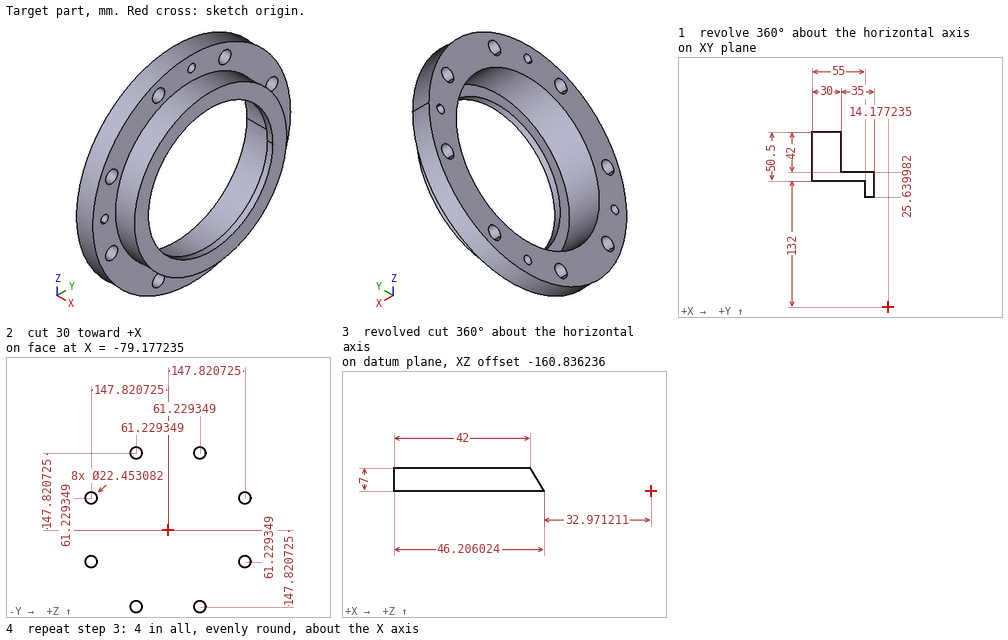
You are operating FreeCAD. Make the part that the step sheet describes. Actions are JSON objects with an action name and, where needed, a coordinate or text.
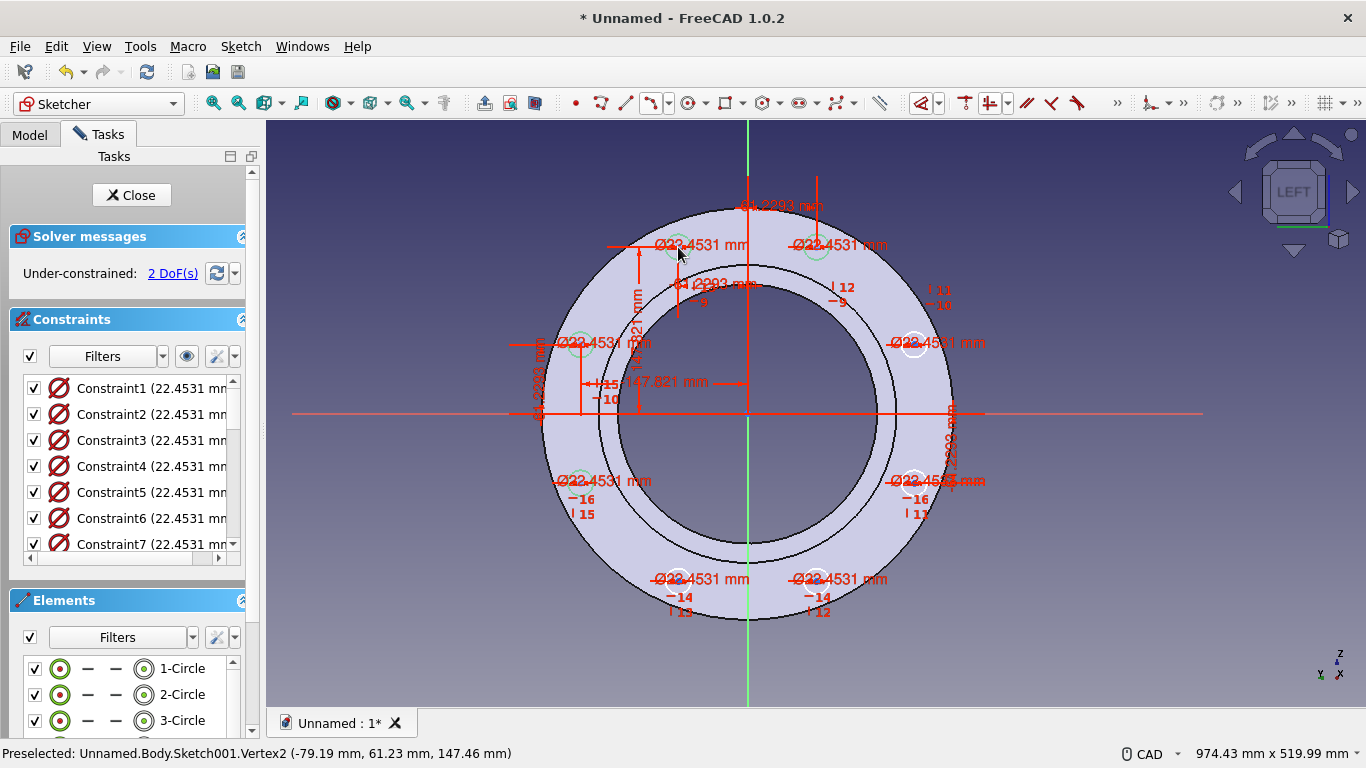
{"action": "left_click", "coordinate": [914, 345]}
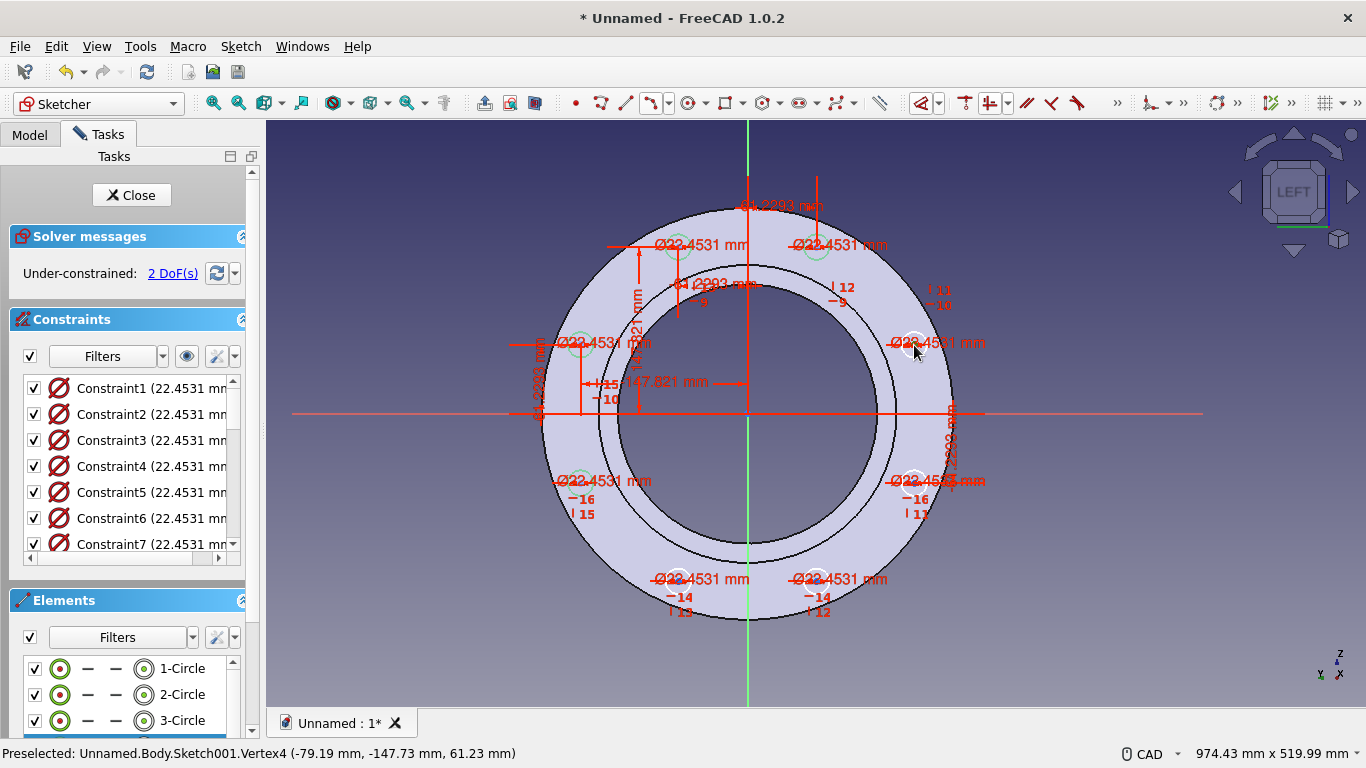
{"action": "key", "text": "l"}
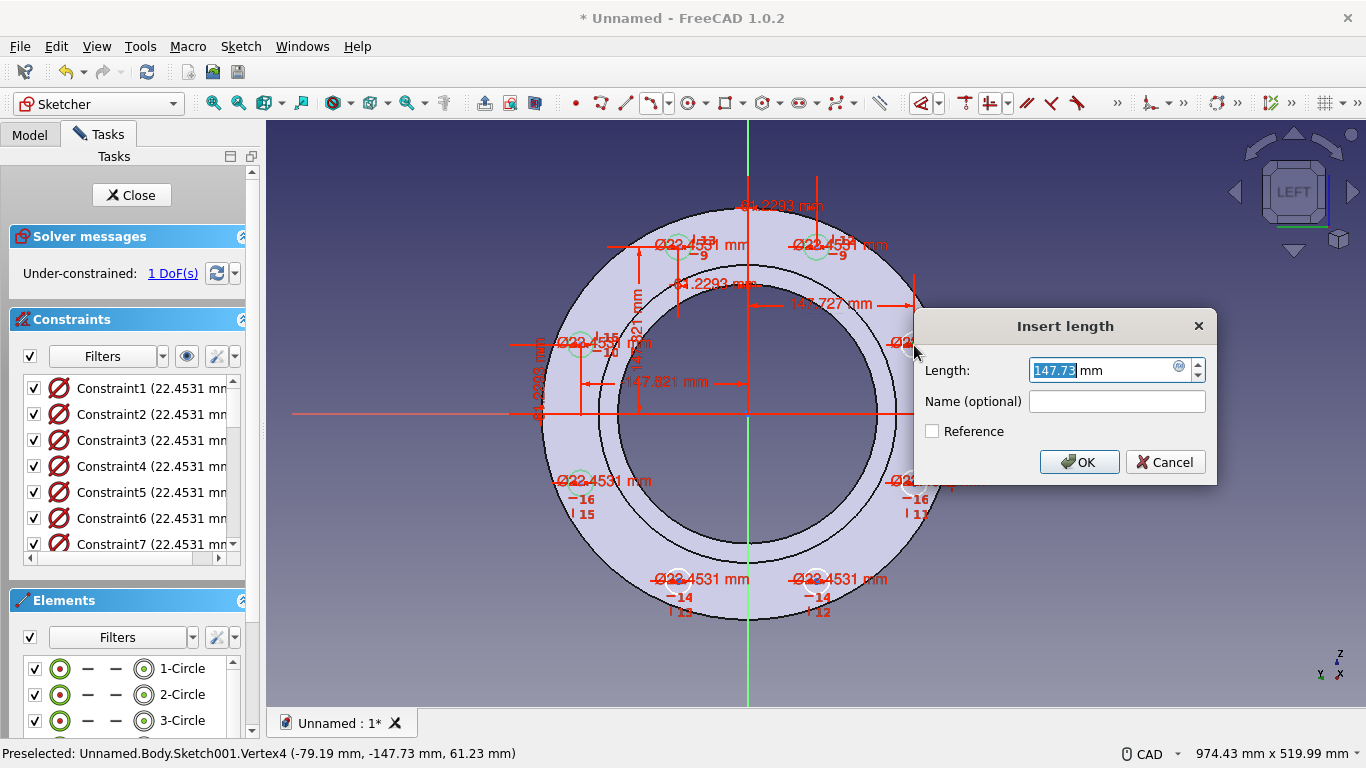
{"action": "type", "text": "147.820725"}
{"action": "key", "text": "Return"}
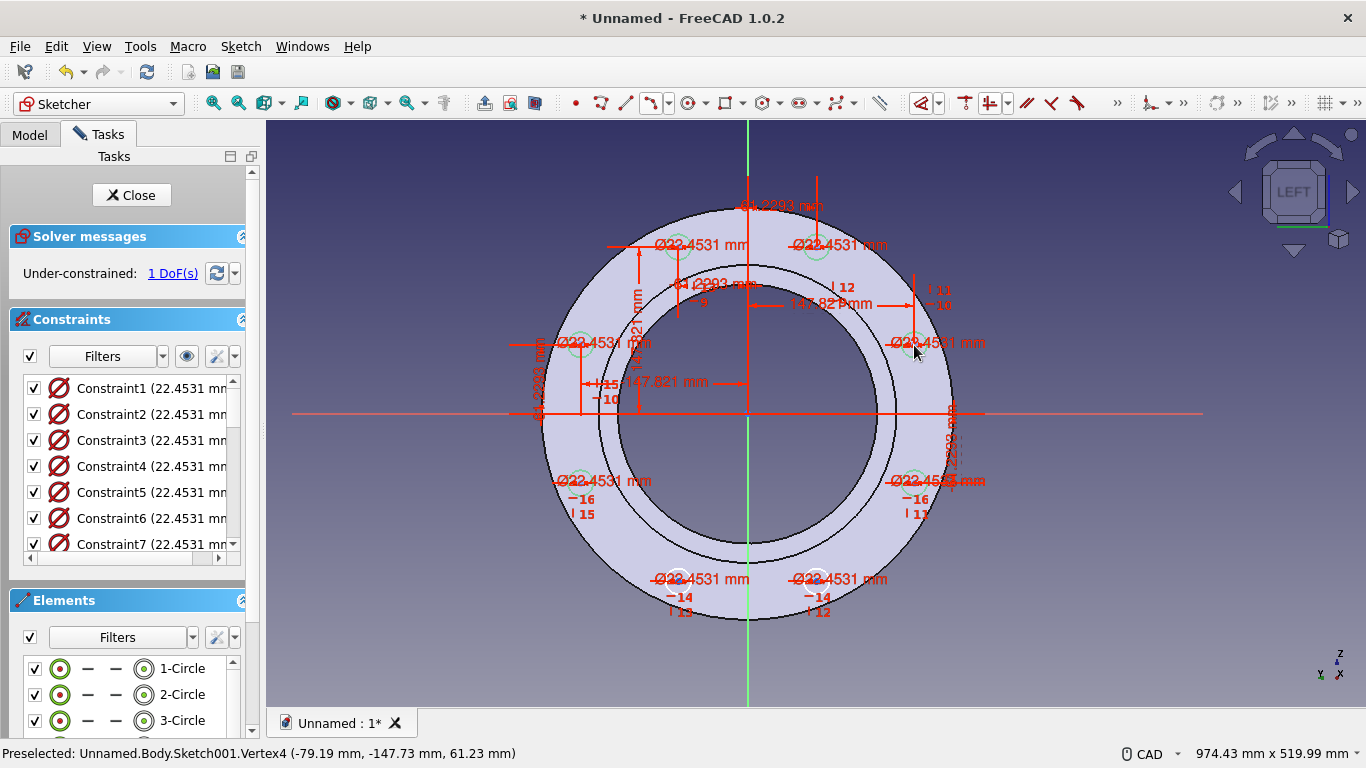
{"action": "left_click", "coordinate": [817, 581]}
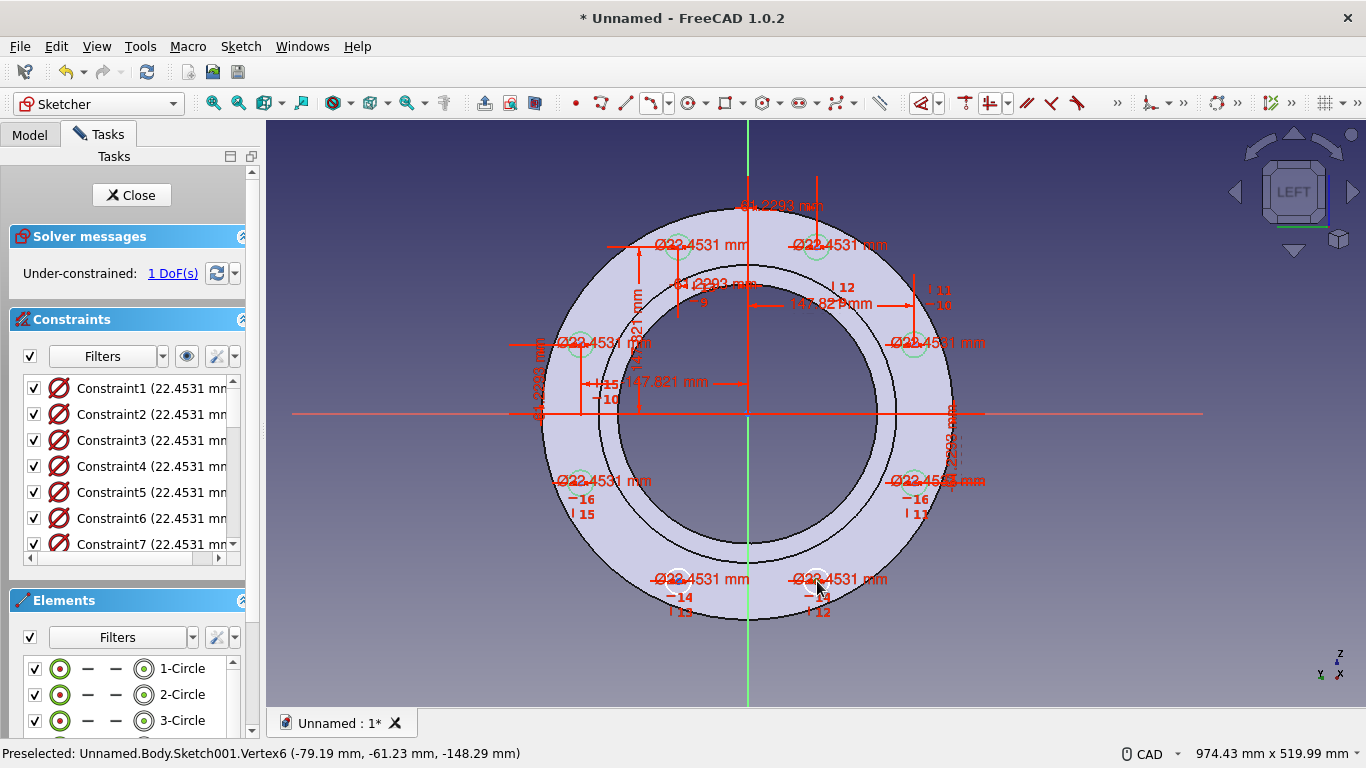
{"action": "key", "text": "i"}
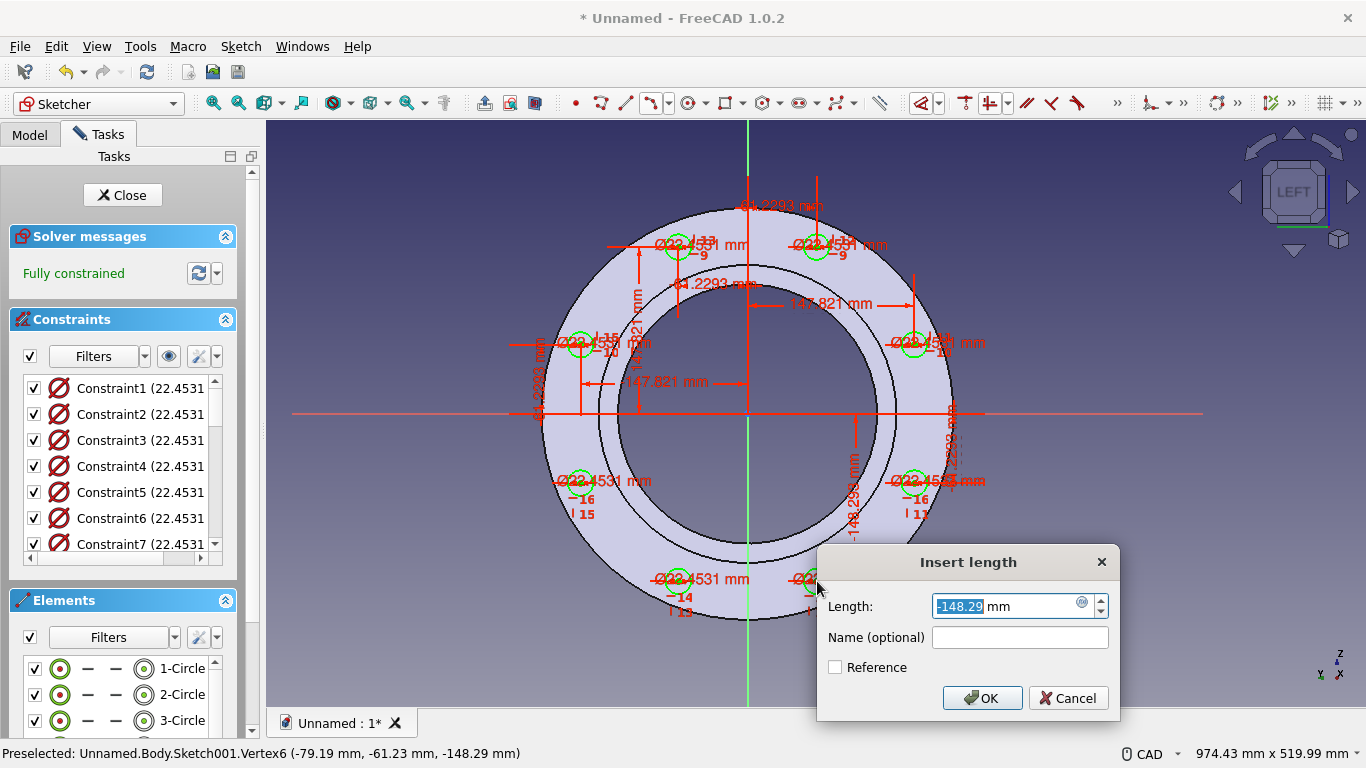
{"action": "type", "text": "-147.820725"}
{"action": "key", "text": "Return"}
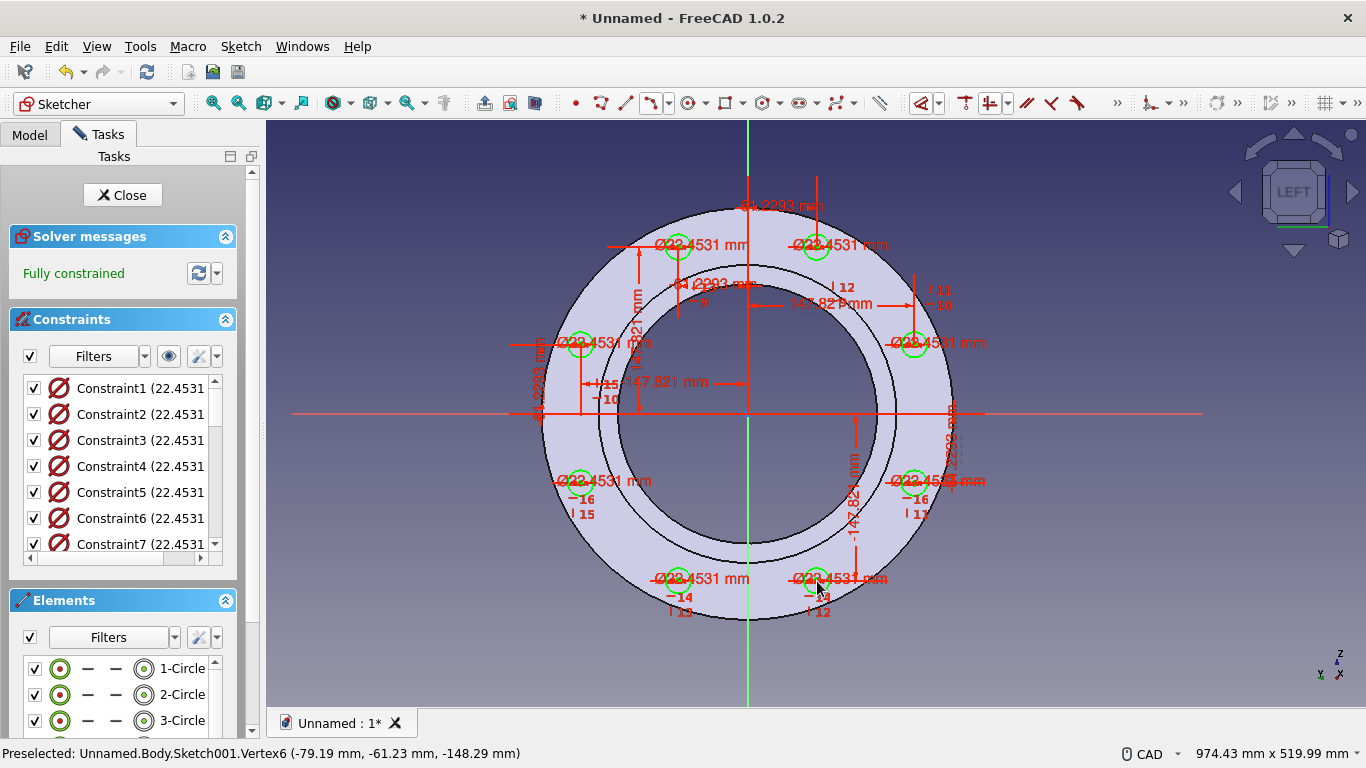
{"action": "left_click", "coordinate": [123, 195]}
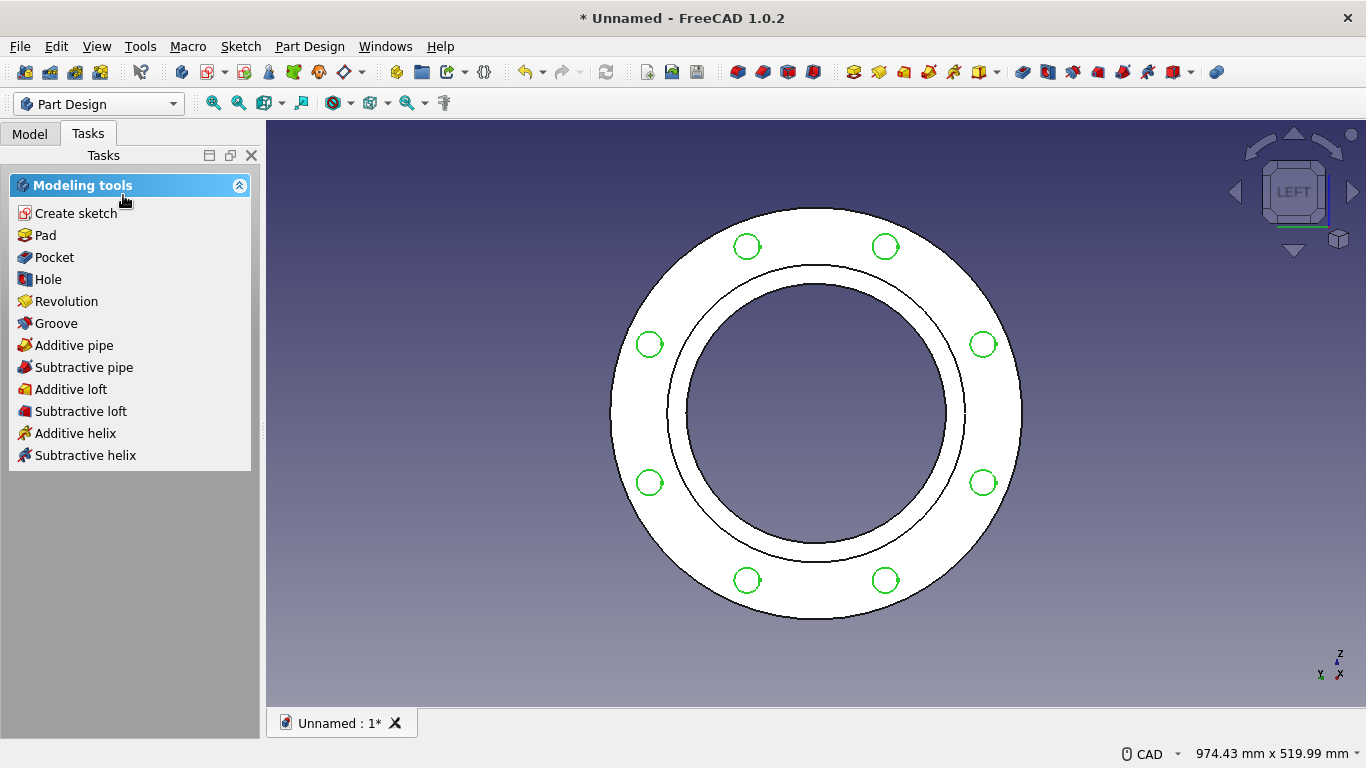
{"action": "left_click", "coordinate": [1023, 72]}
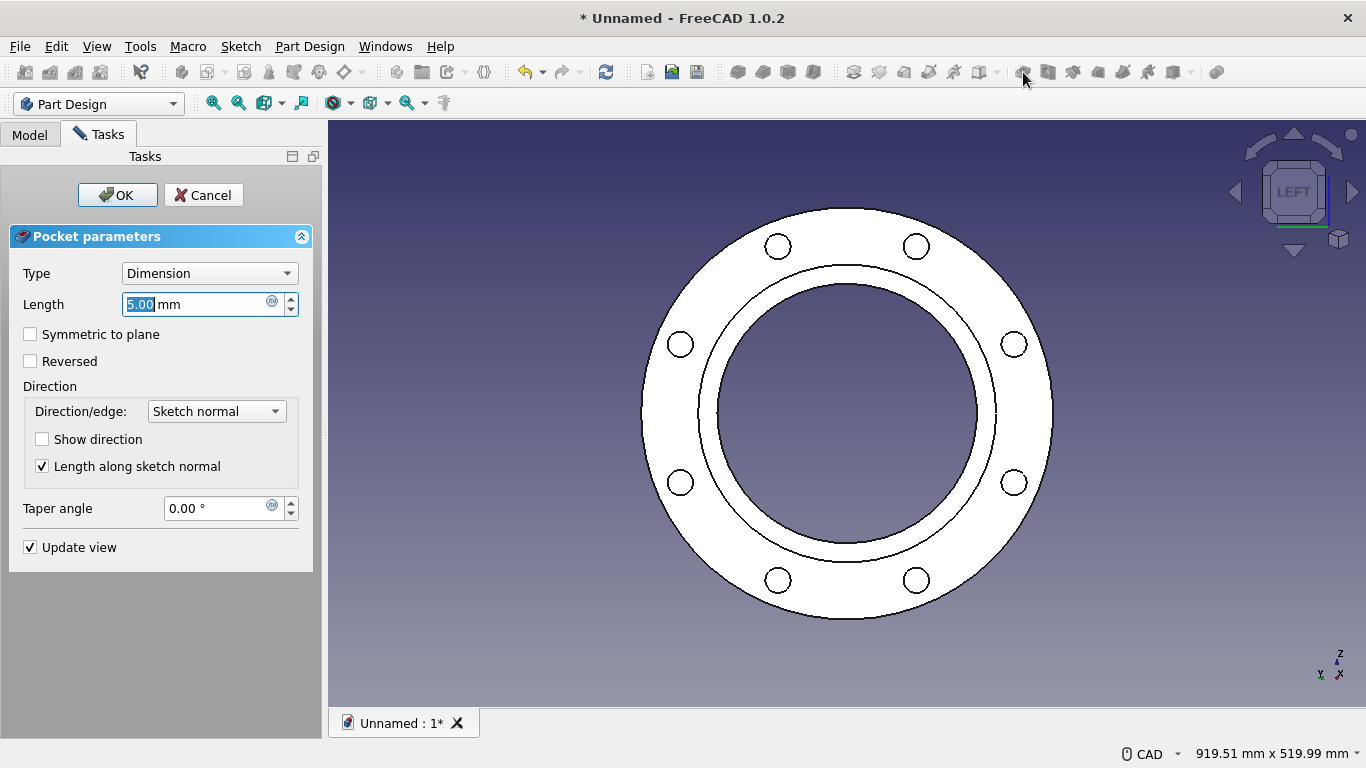
{"action": "type", "text": "30"}
{"action": "key", "text": "Tab"}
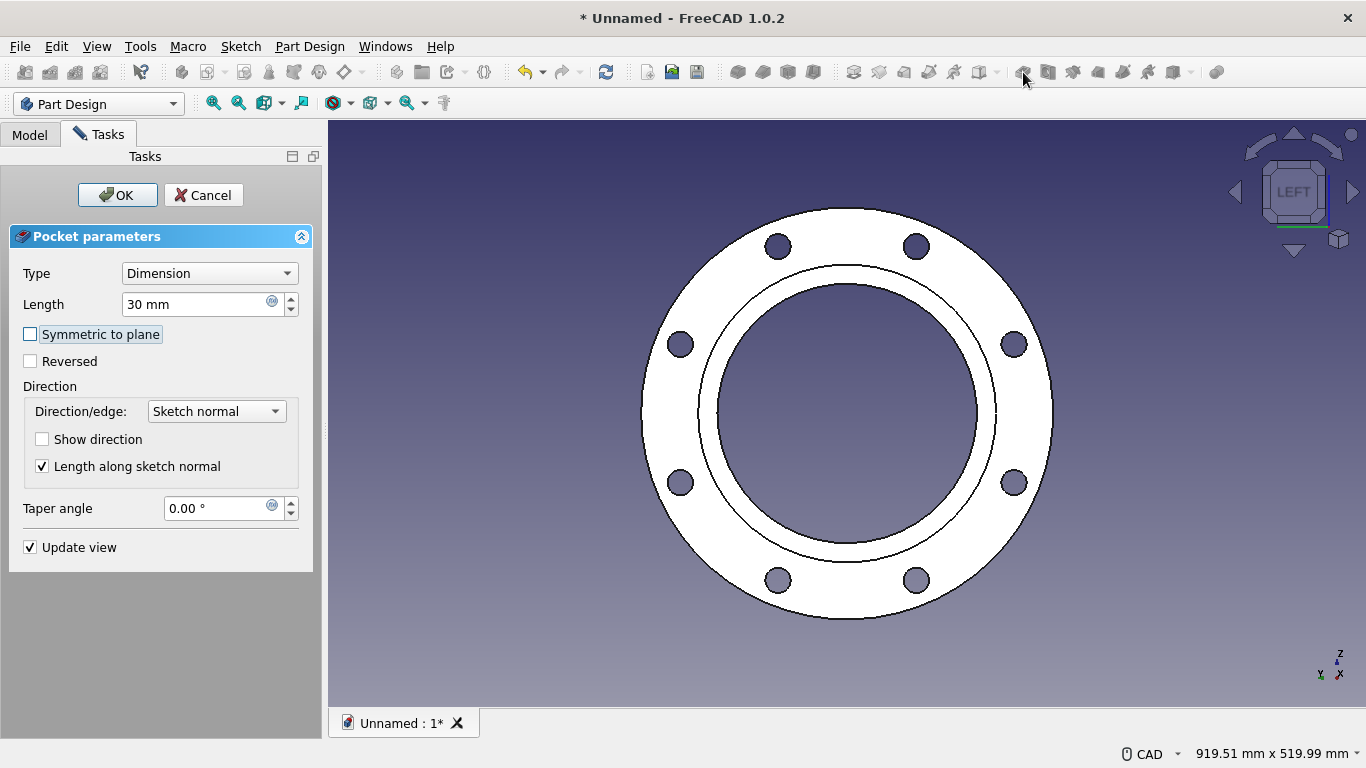
{"action": "left_click", "coordinate": [118, 195]}